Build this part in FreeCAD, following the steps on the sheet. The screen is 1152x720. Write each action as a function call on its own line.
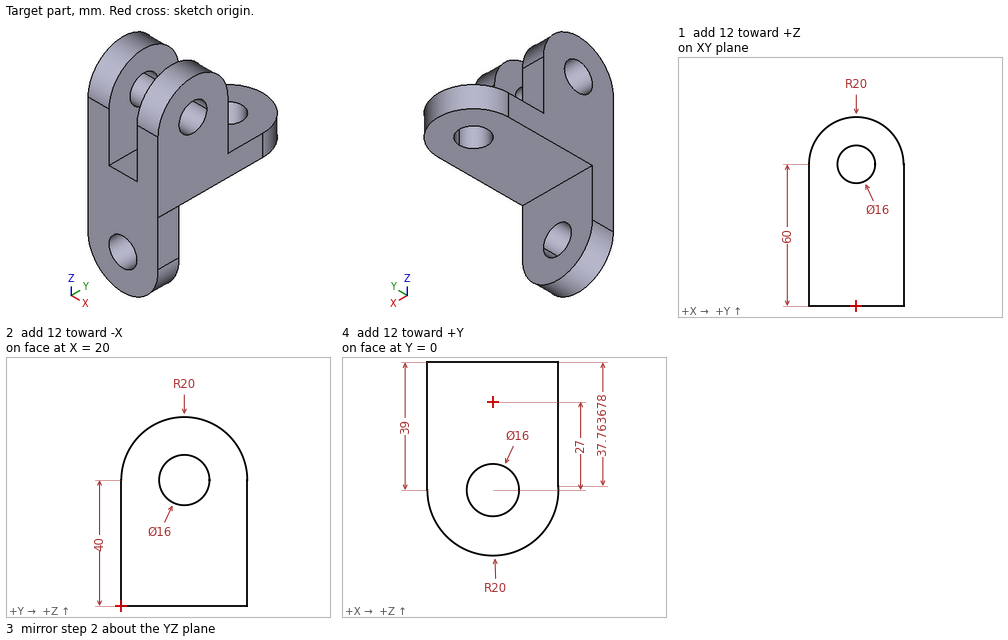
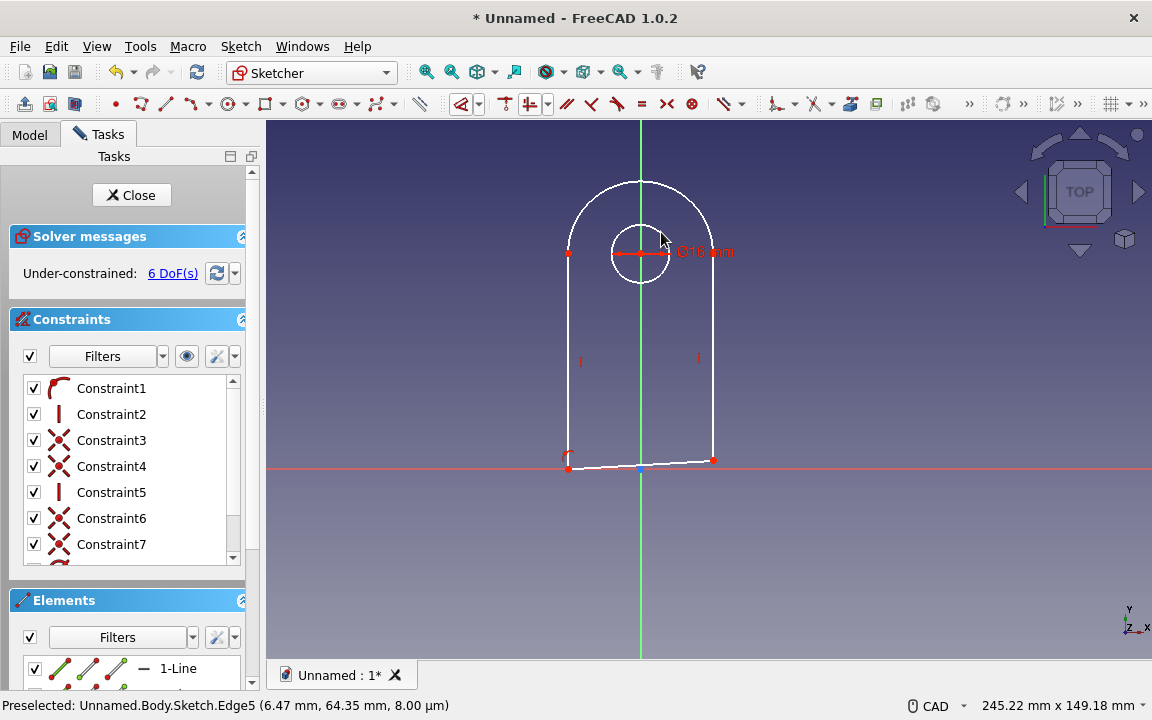
click(568, 319)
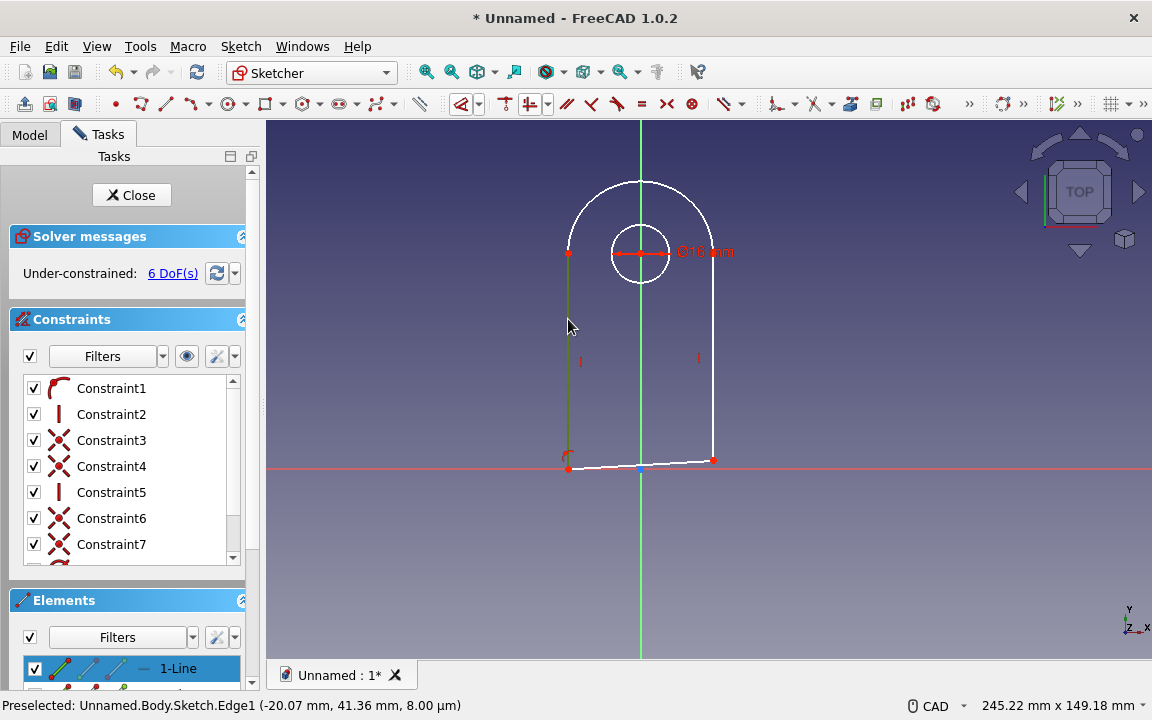
click(683, 195)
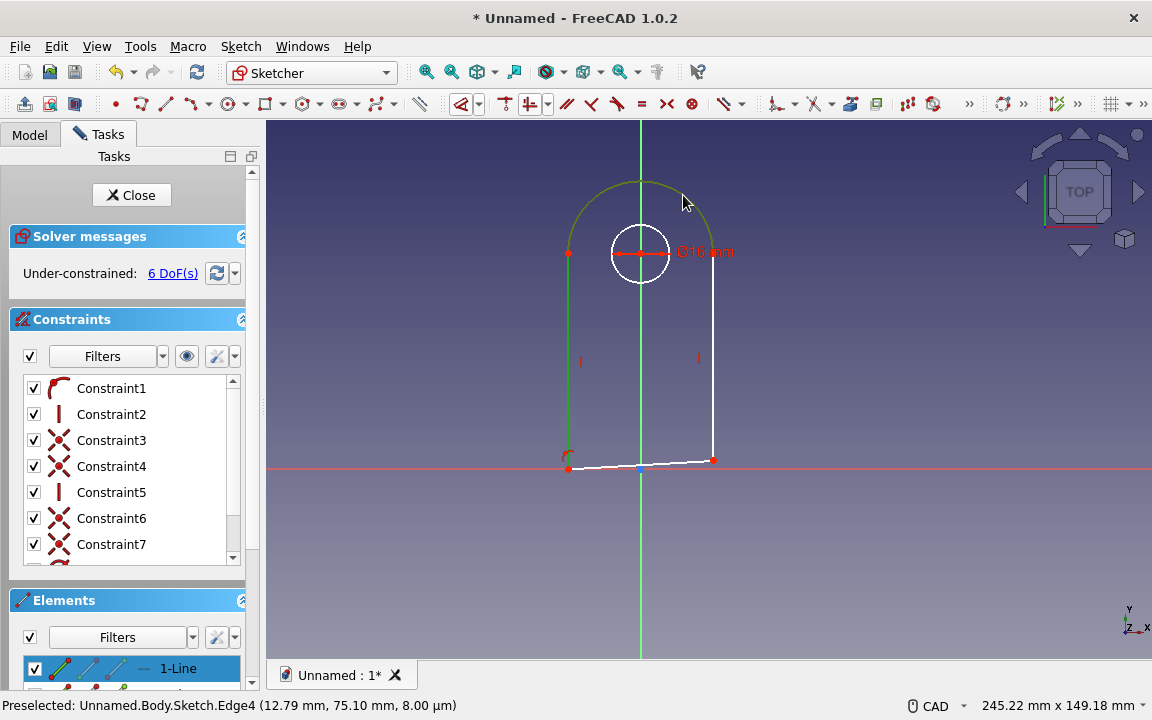
key(t)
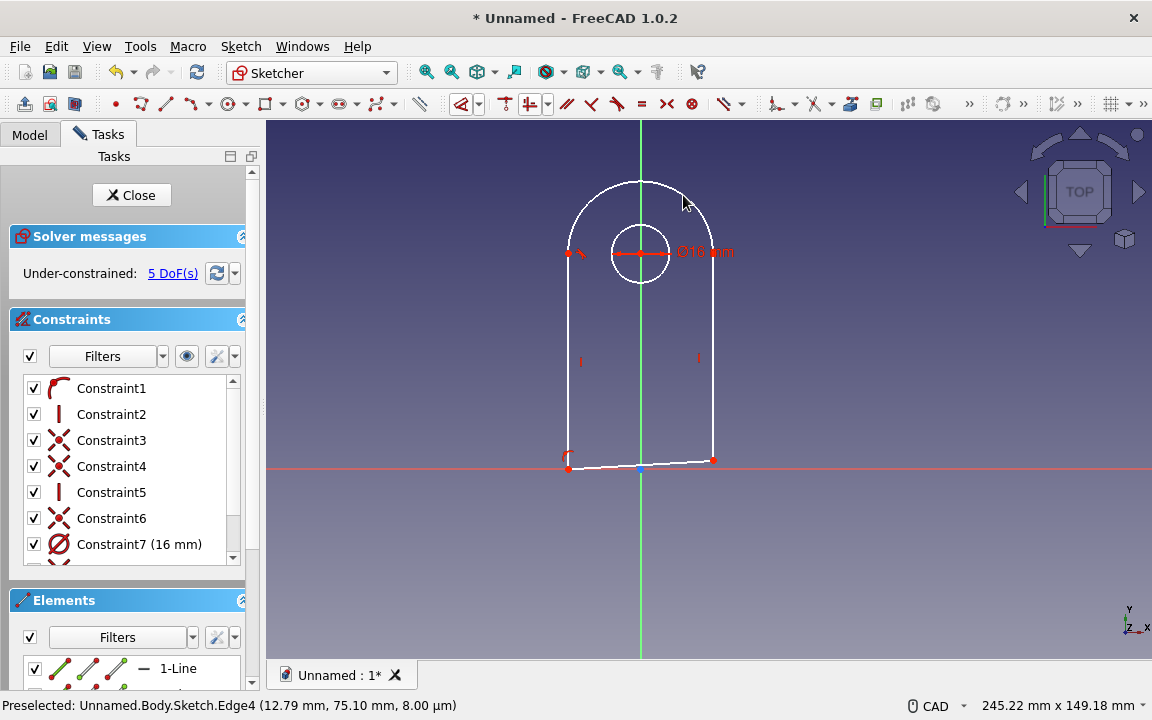
click(713, 399)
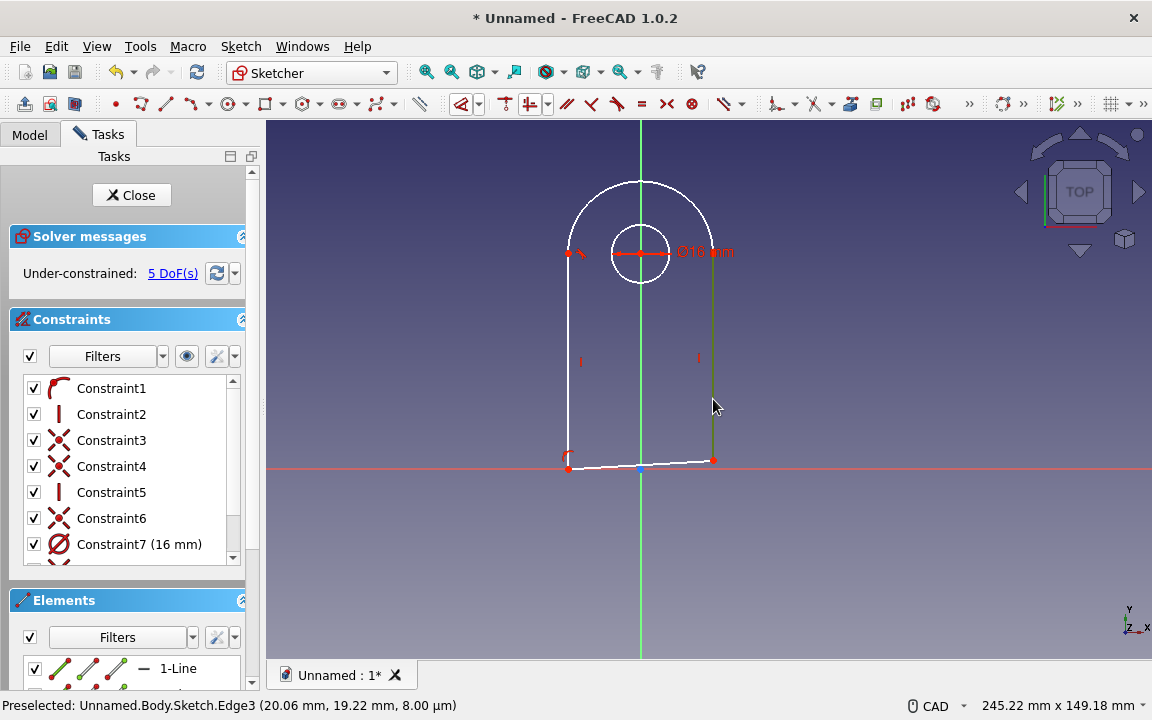
click(683, 195)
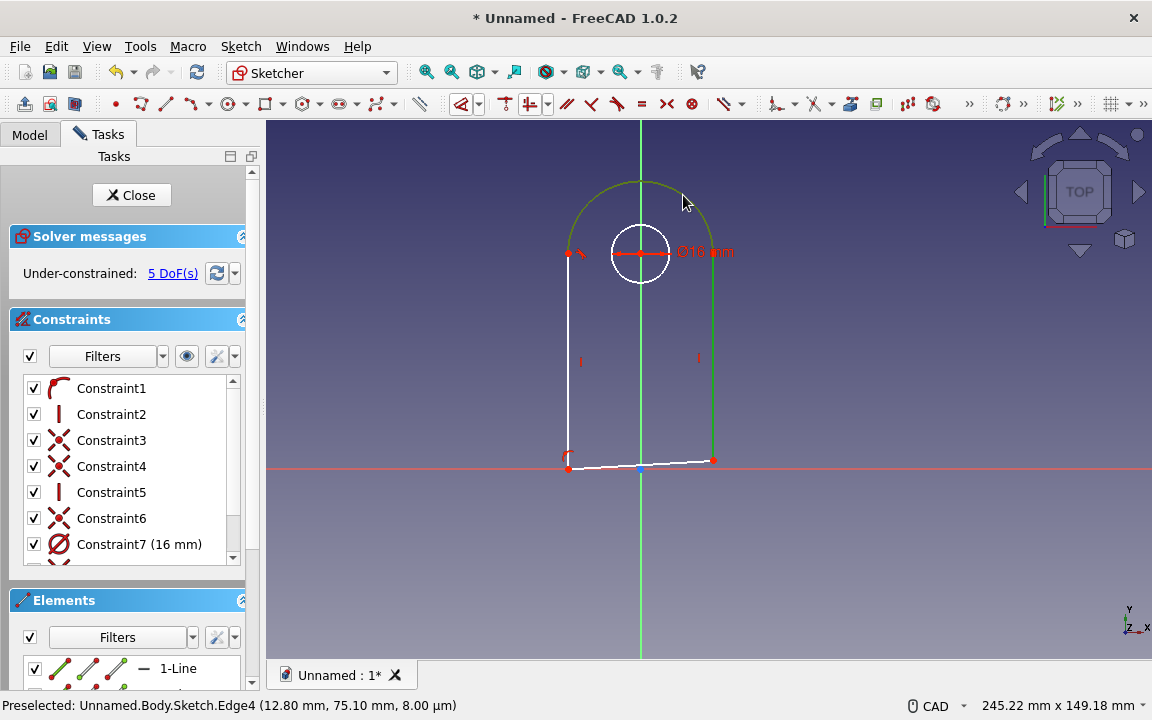
key(t)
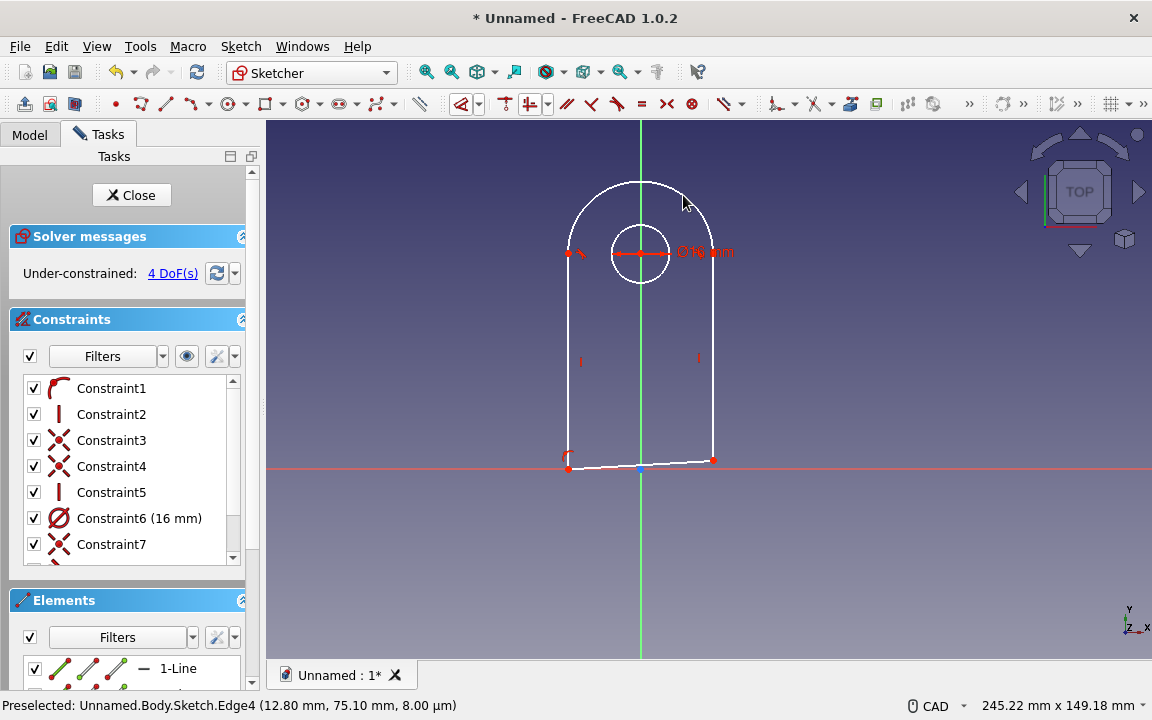
click(612, 467)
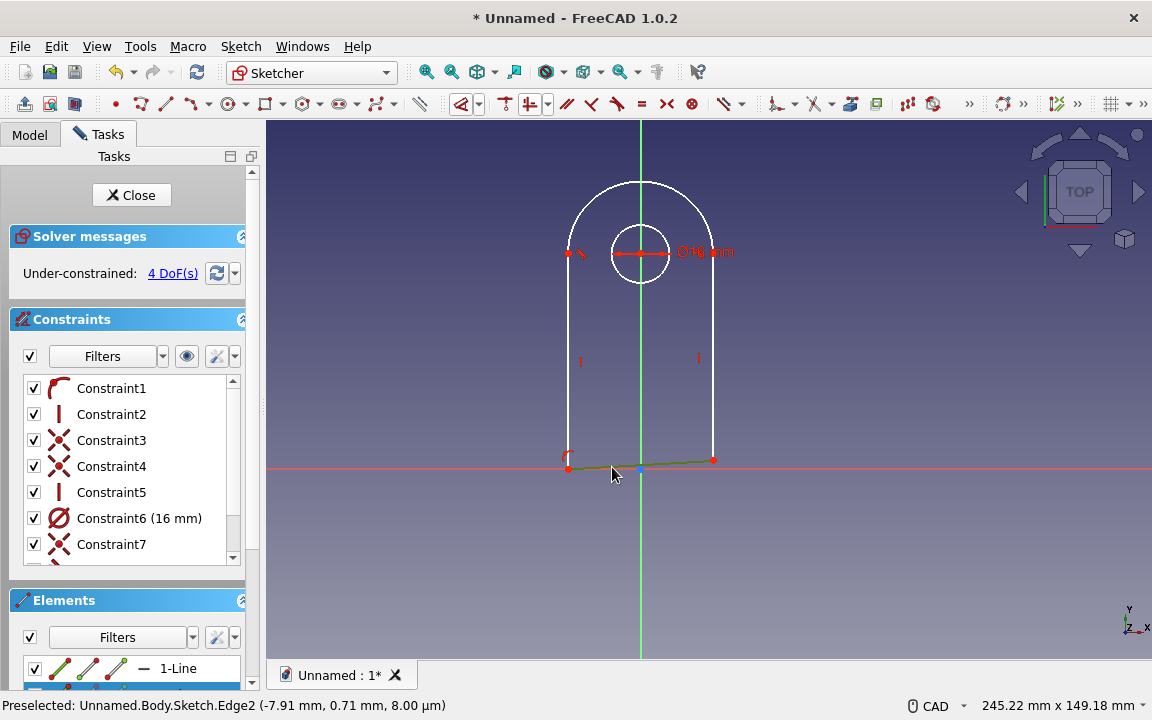
click(548, 104)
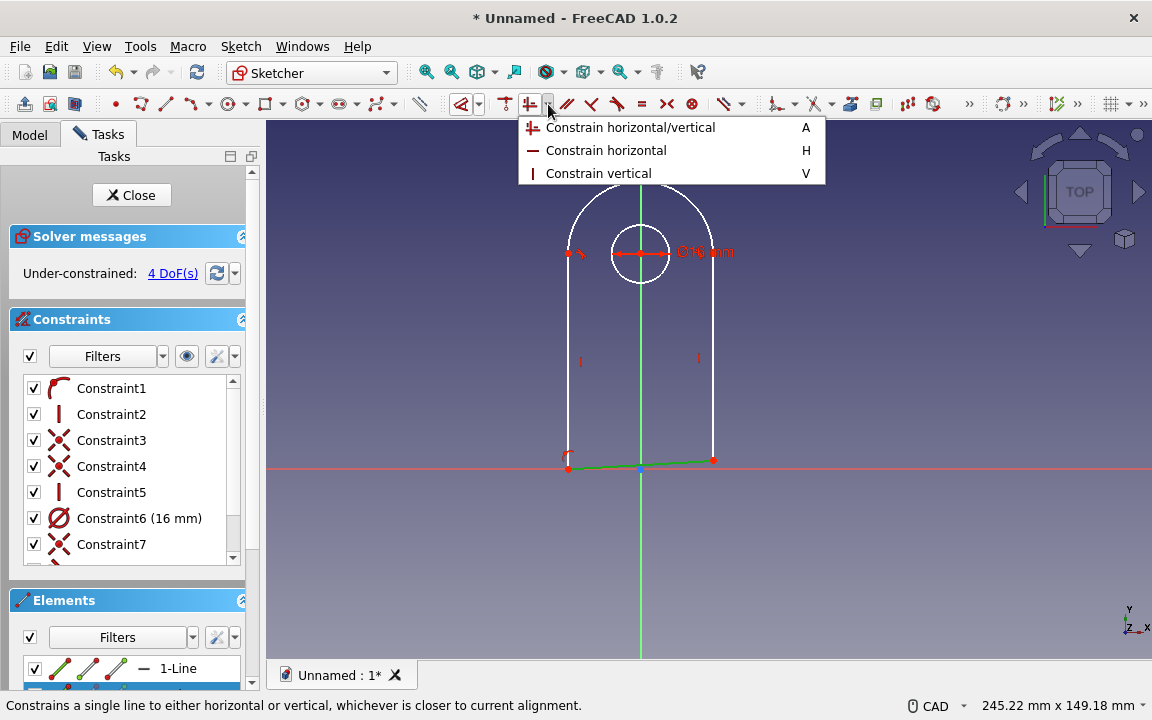
click(672, 150)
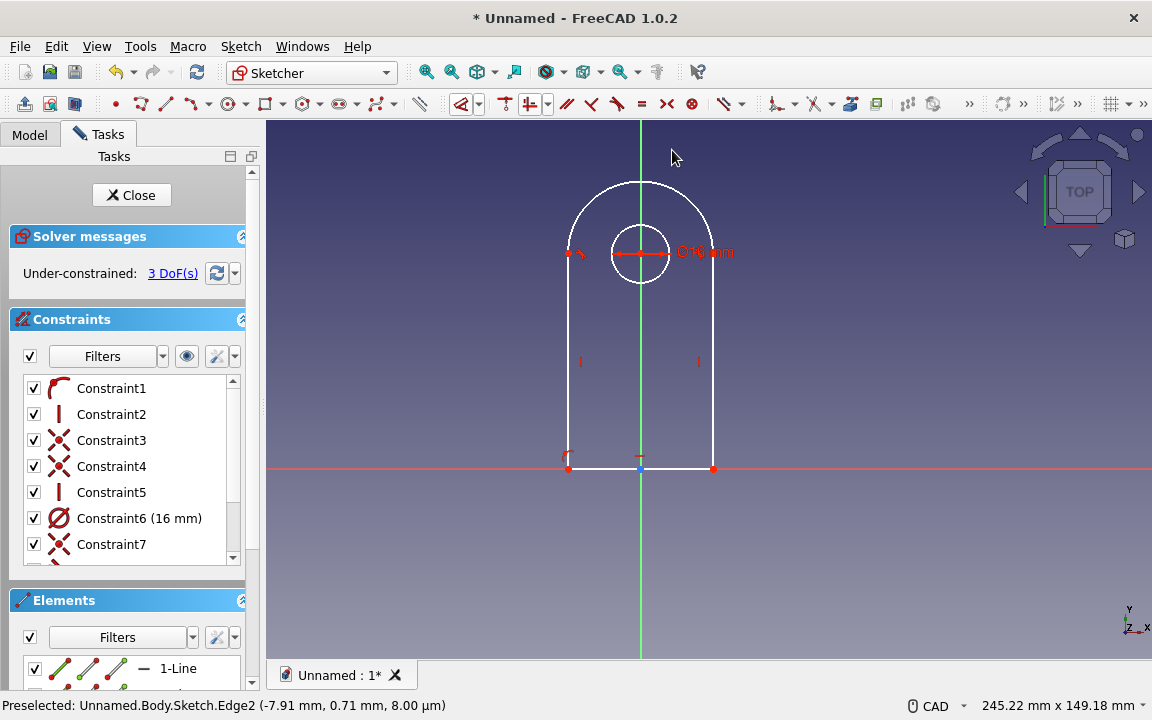
click(641, 254)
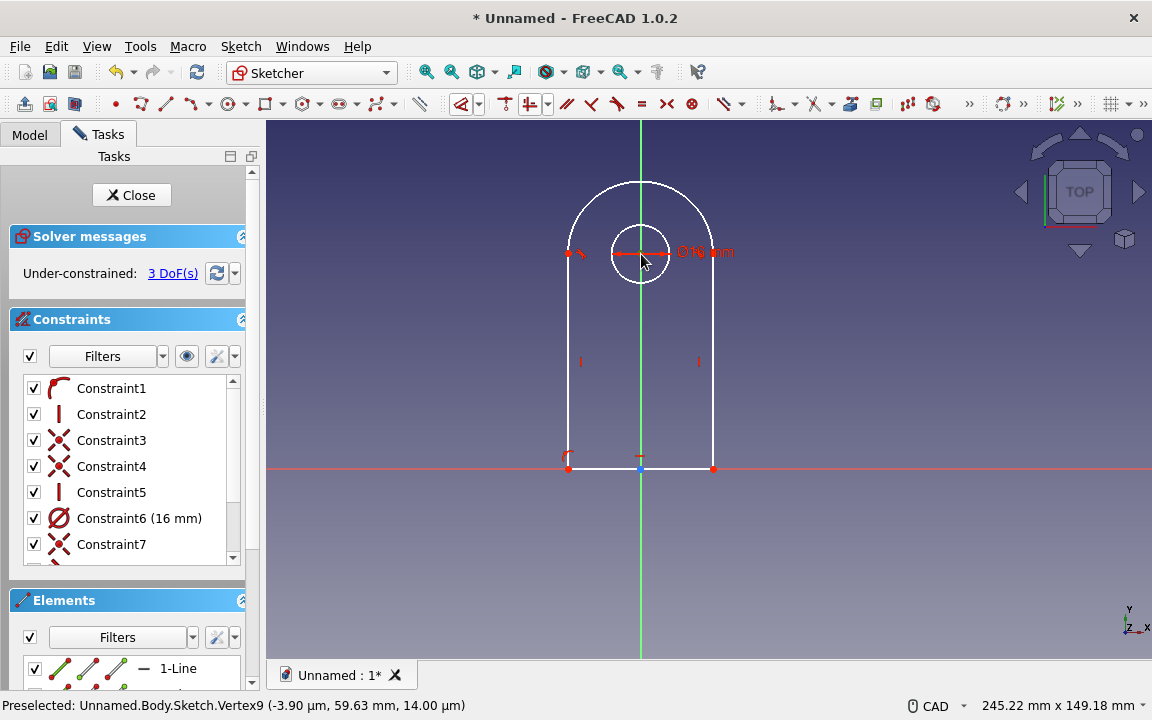
click(641, 596)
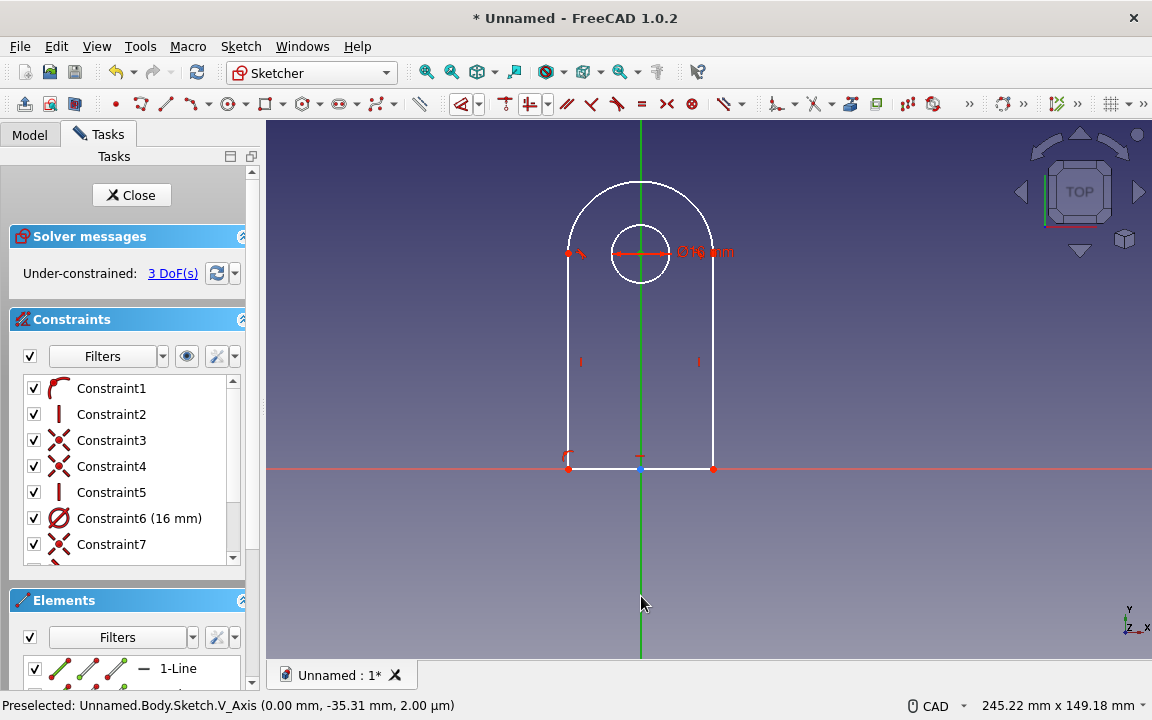
key(c)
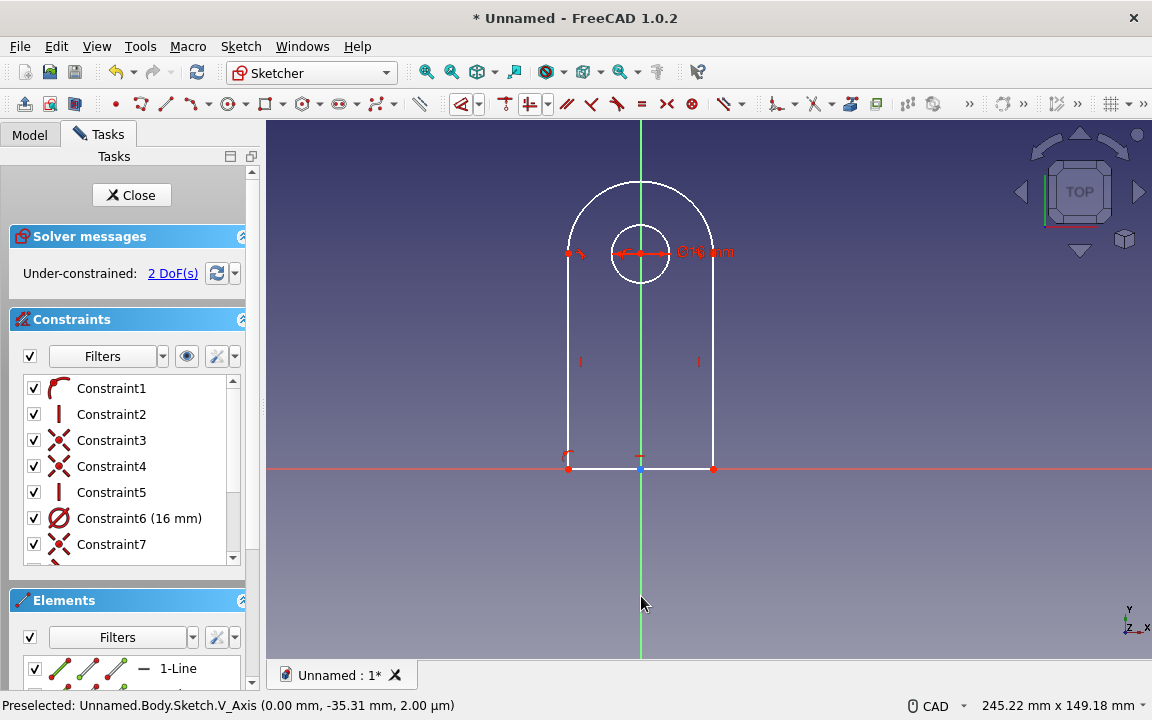
click(460, 104)